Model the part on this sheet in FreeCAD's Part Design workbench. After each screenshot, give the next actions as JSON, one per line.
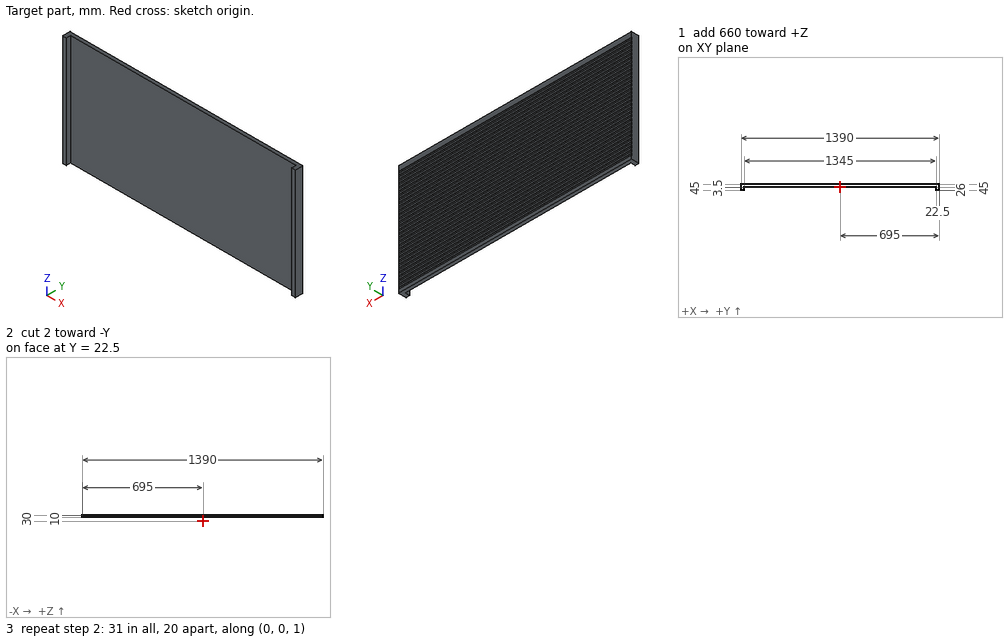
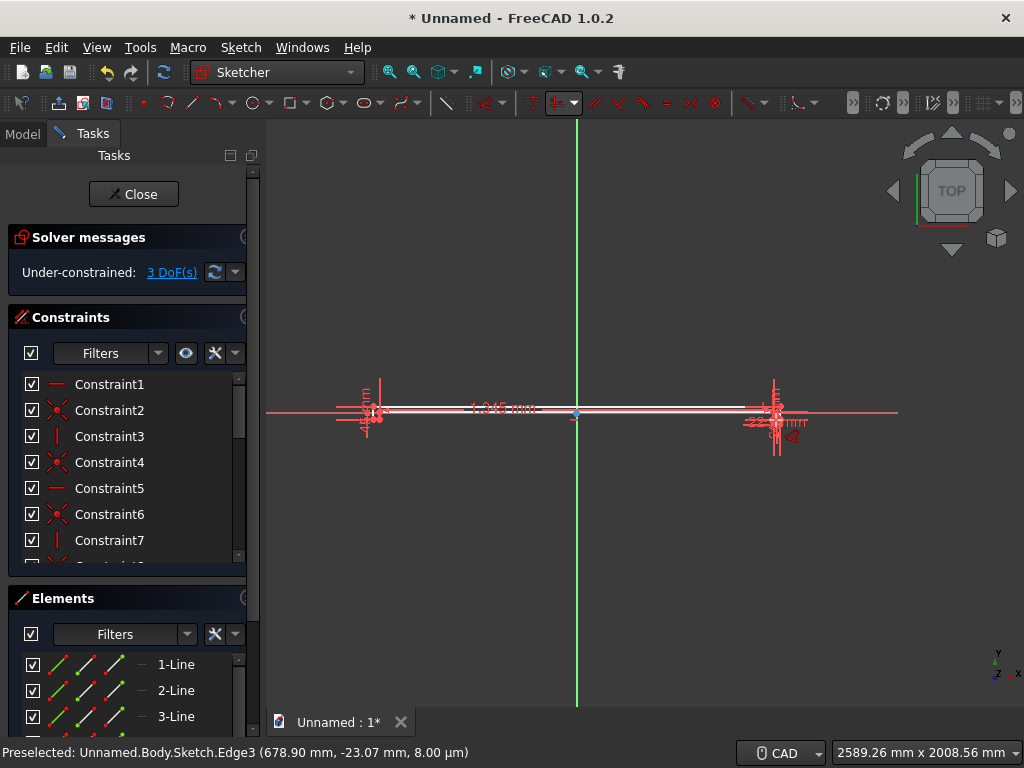
{"action": "scroll", "coordinate": [658, 407], "scroll_direction": "up", "scroll_amount": 5}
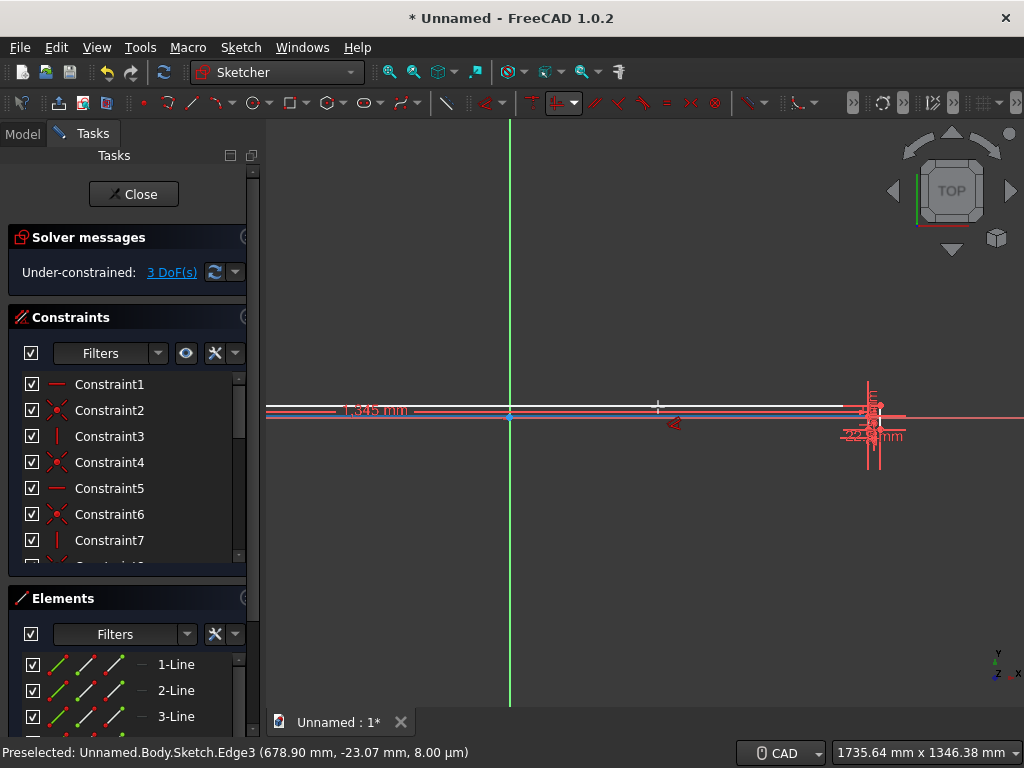
{"action": "left_click", "coordinate": [657, 405]}
{"action": "left_click", "coordinate": [576, 371]}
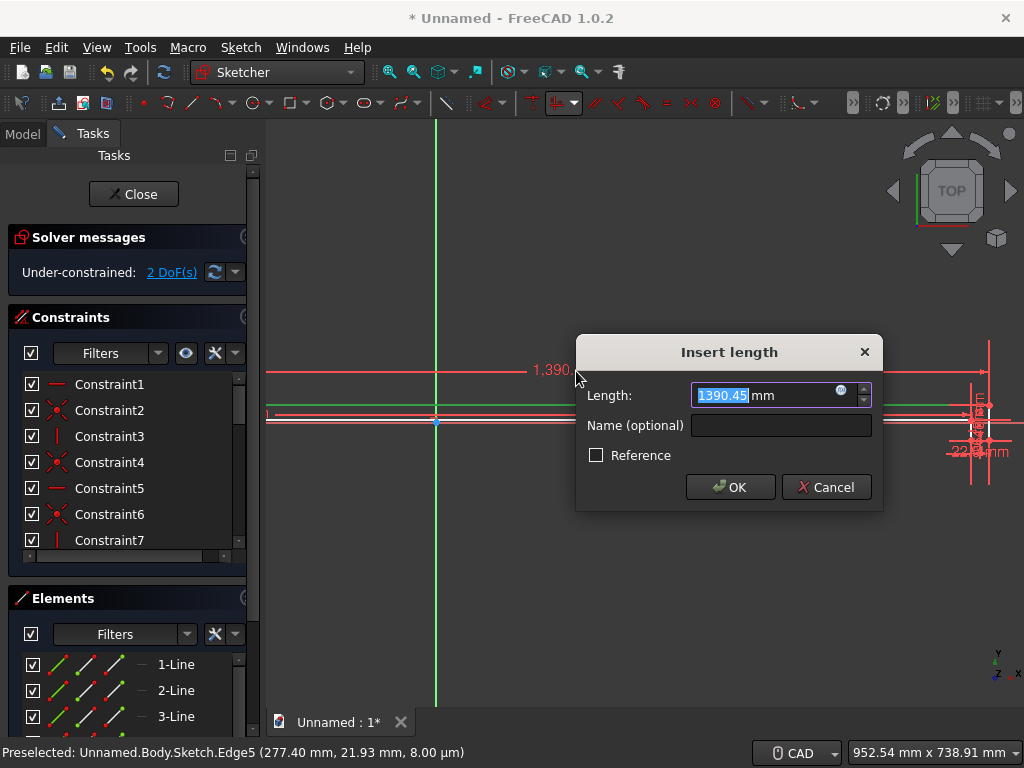
{"action": "type", "text": "1390"}
{"action": "key", "text": "Return"}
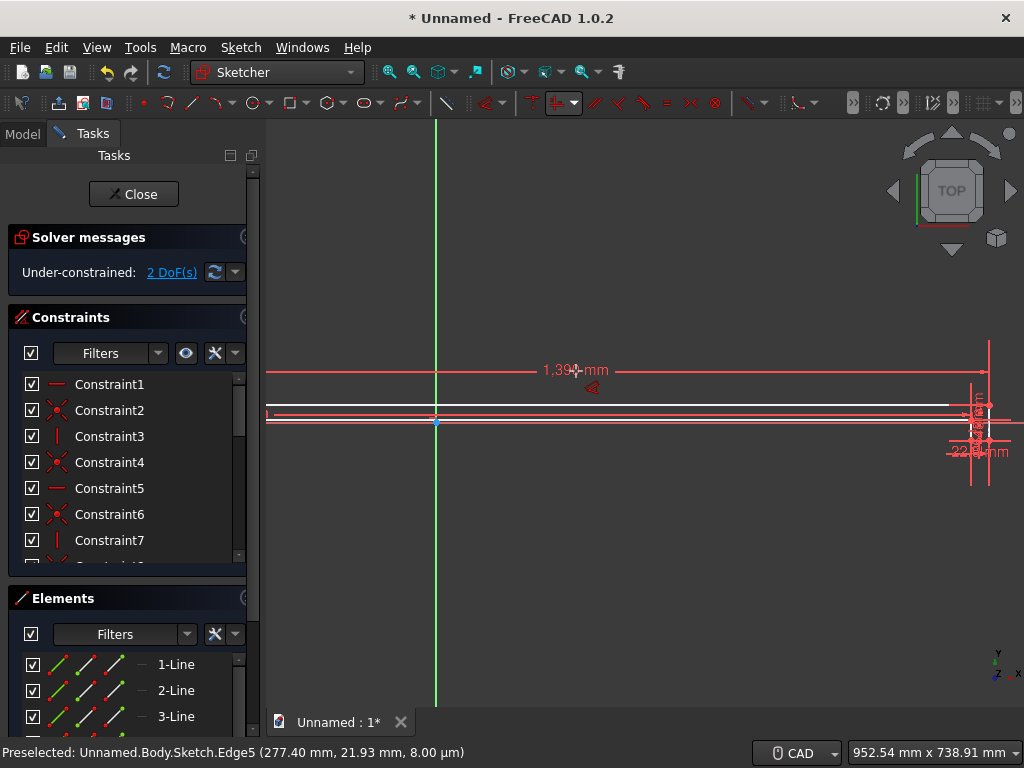
{"action": "scroll", "coordinate": [658, 407], "scroll_direction": "down", "scroll_amount": 5}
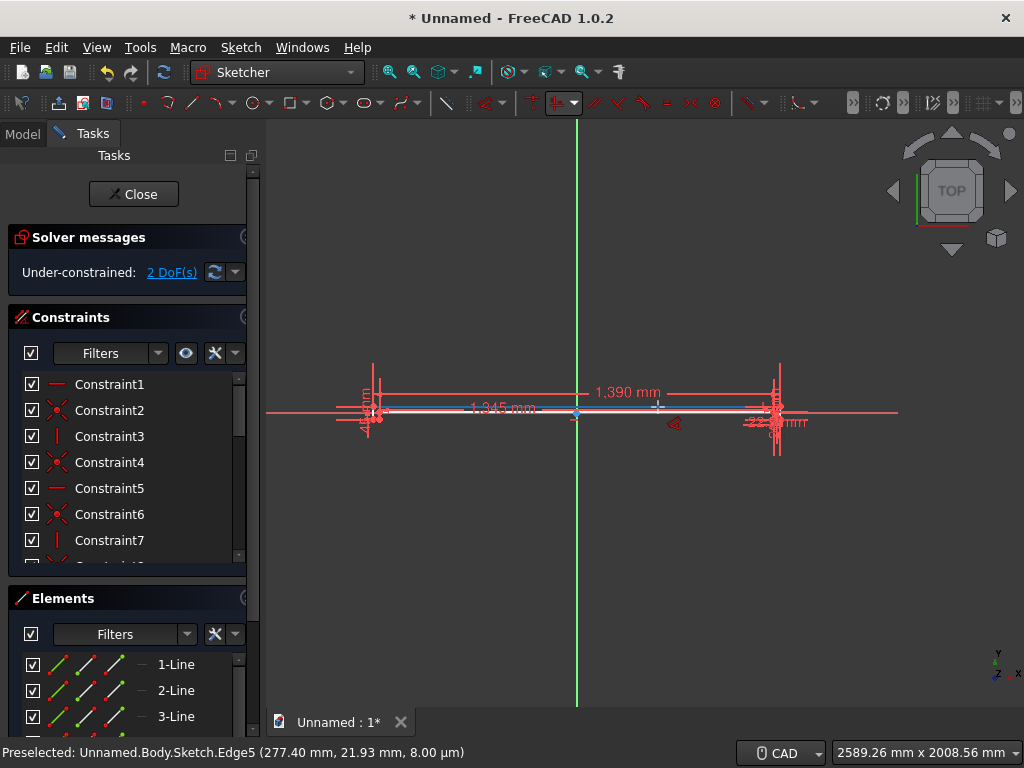
{"action": "scroll", "coordinate": [380, 412], "scroll_direction": "up", "scroll_amount": 19}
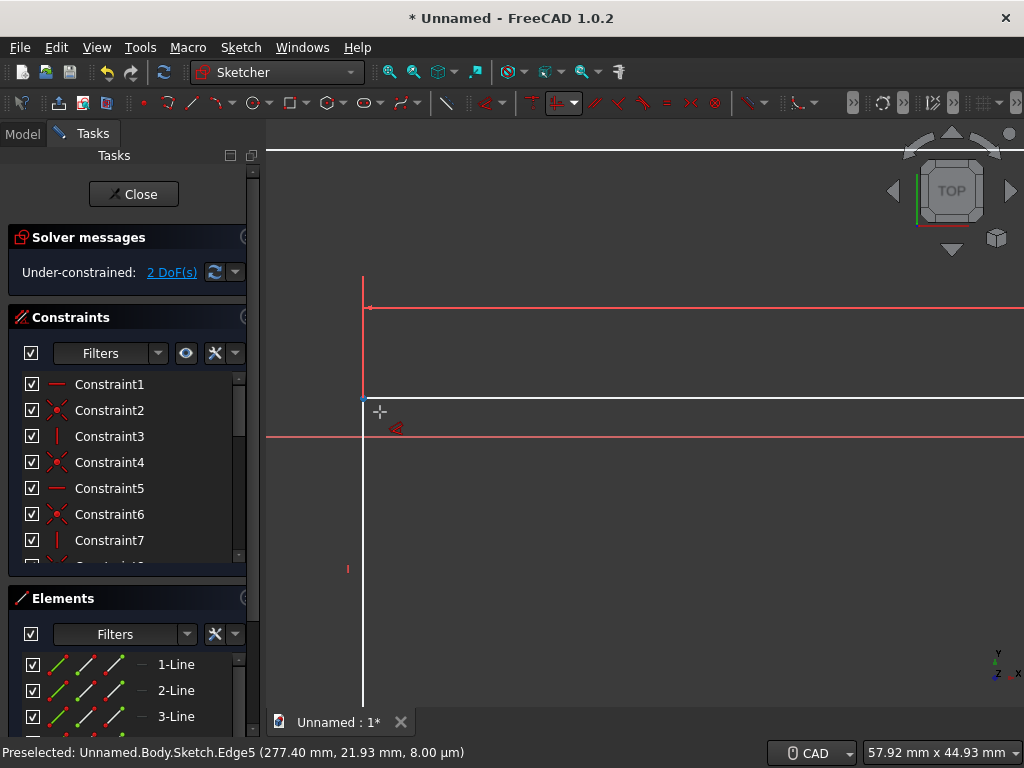
{"action": "left_click", "coordinate": [363, 398]}
{"action": "left_click", "coordinate": [329, 417]}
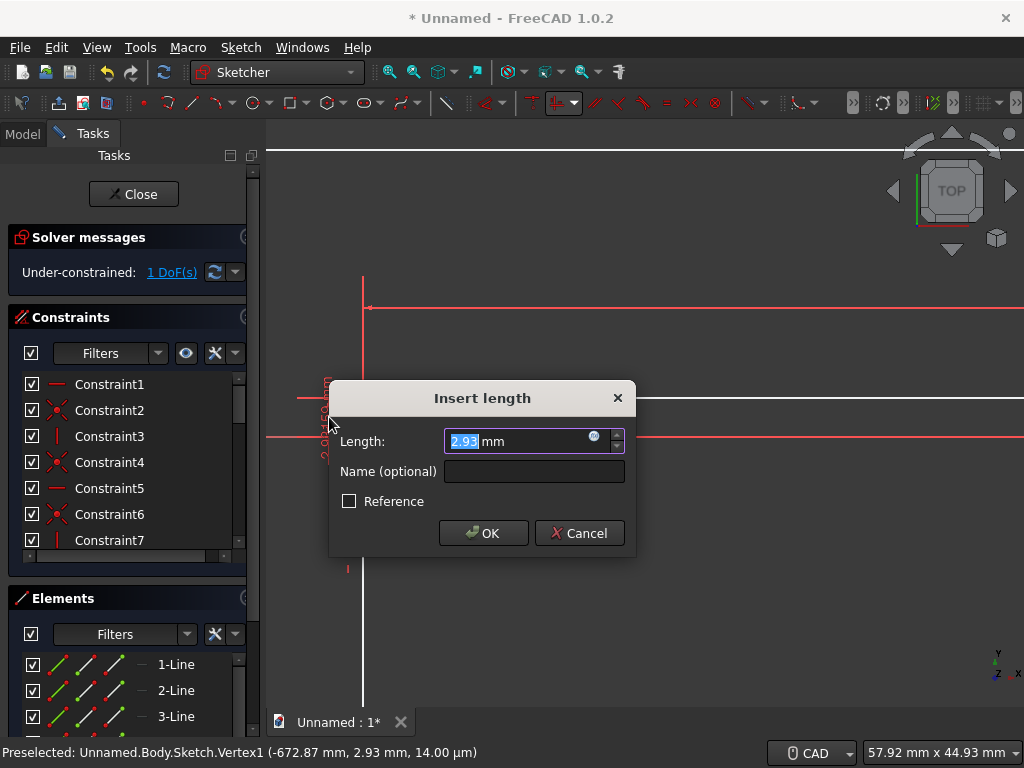
{"action": "type", "text": "3.5"}
{"action": "key", "text": "Return"}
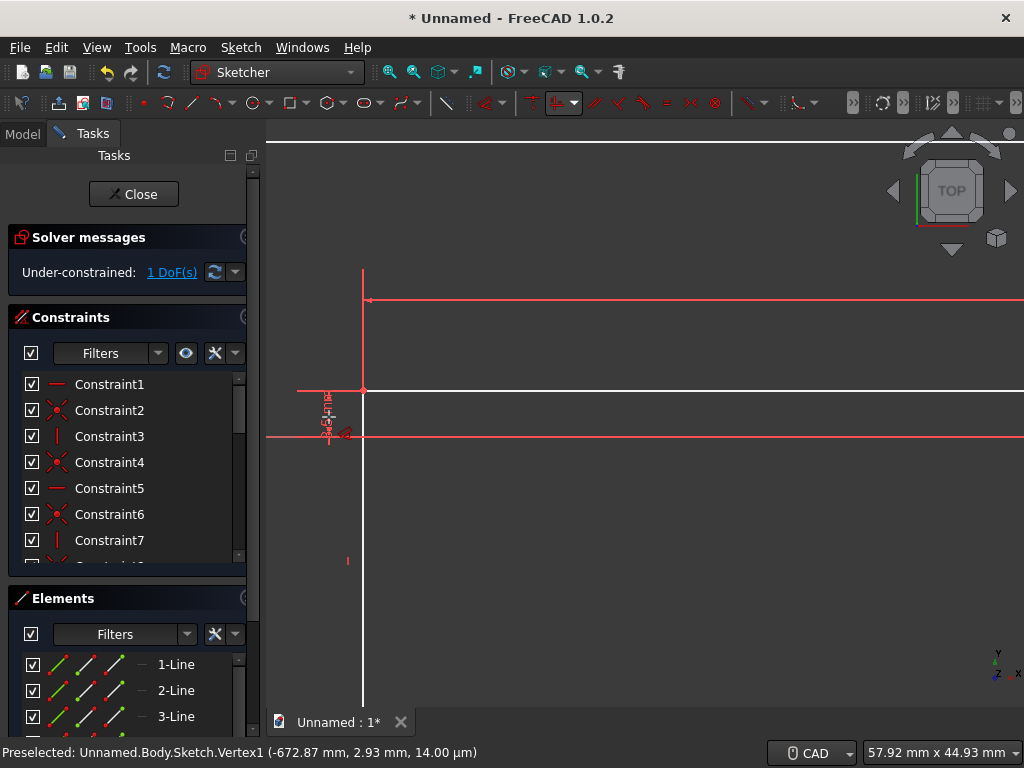
{"action": "scroll", "coordinate": [335, 412], "scroll_direction": "down", "scroll_amount": 18}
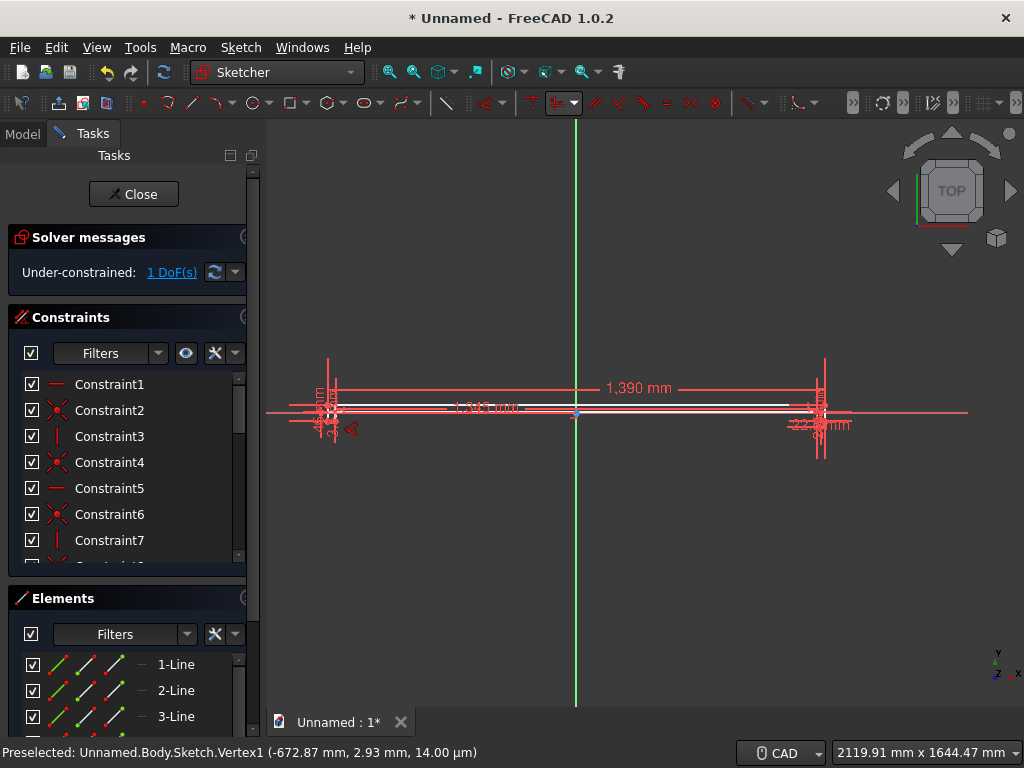
{"action": "scroll", "coordinate": [825, 421], "scroll_direction": "up", "scroll_amount": 3}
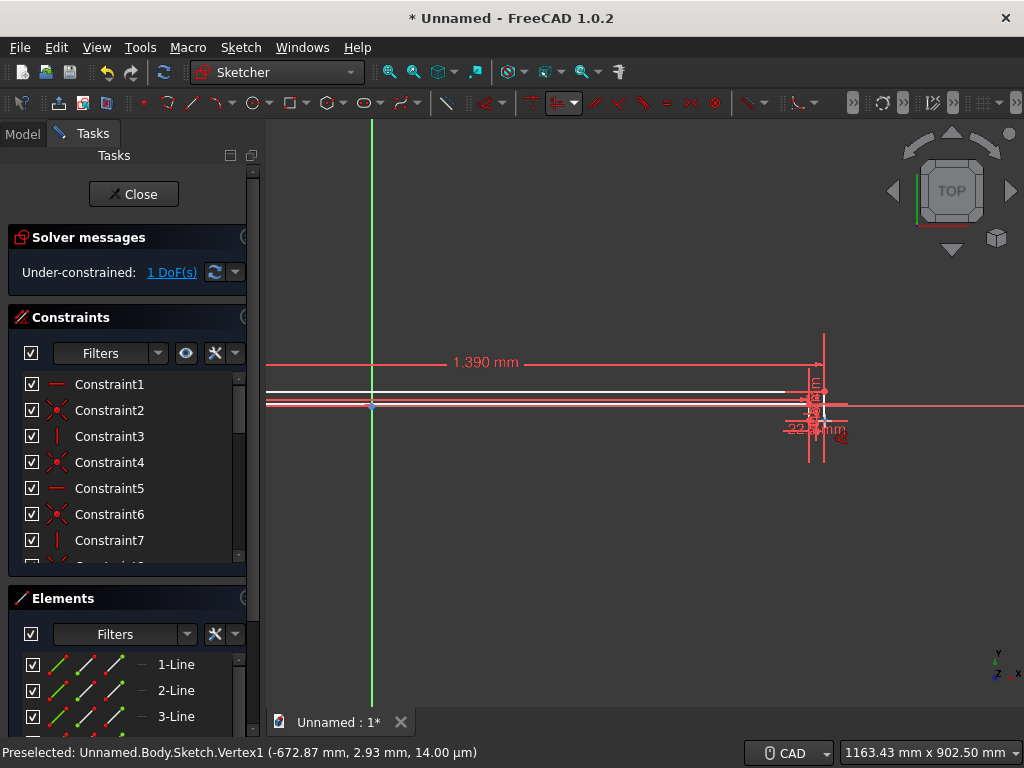
{"action": "left_click", "coordinate": [824, 421]}
{"action": "left_click", "coordinate": [598, 455]}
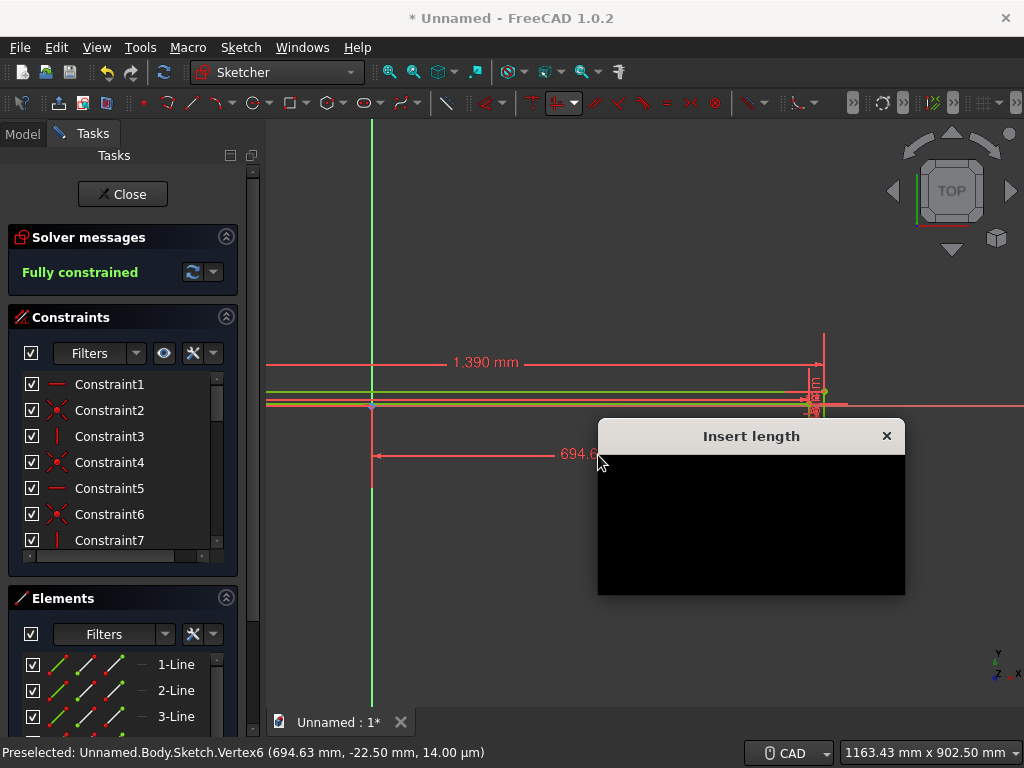
{"action": "type", "text": "695"}
{"action": "key", "text": "Return"}
{"action": "key", "text": "Escape"}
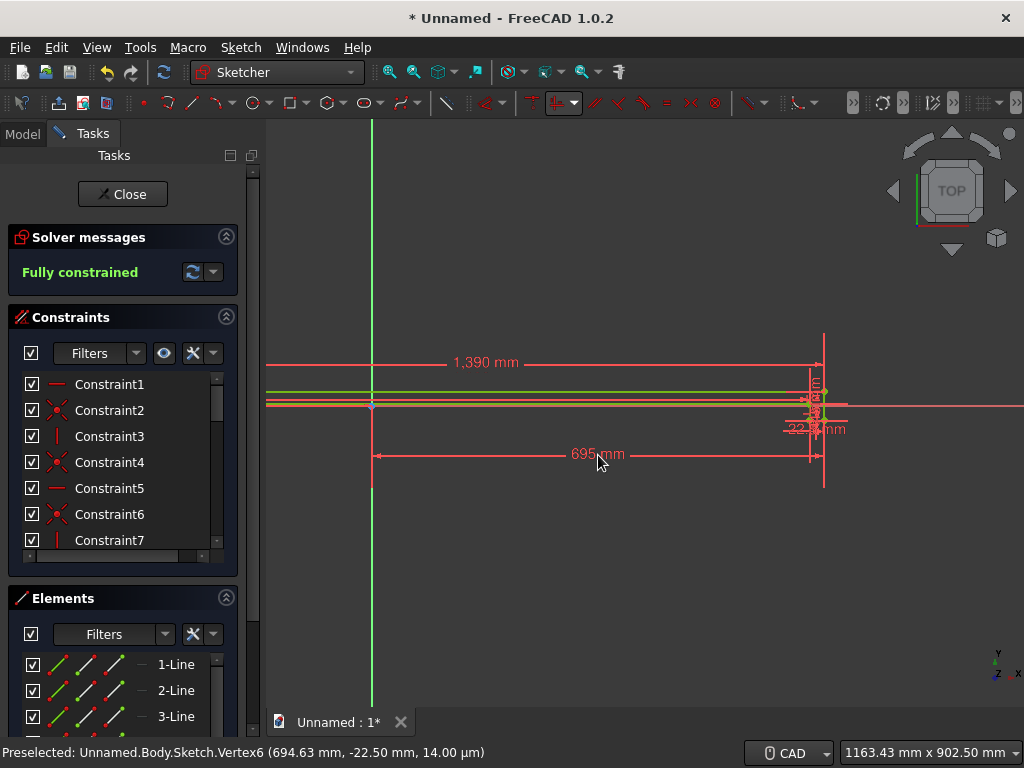
{"action": "left_click", "coordinate": [123, 194]}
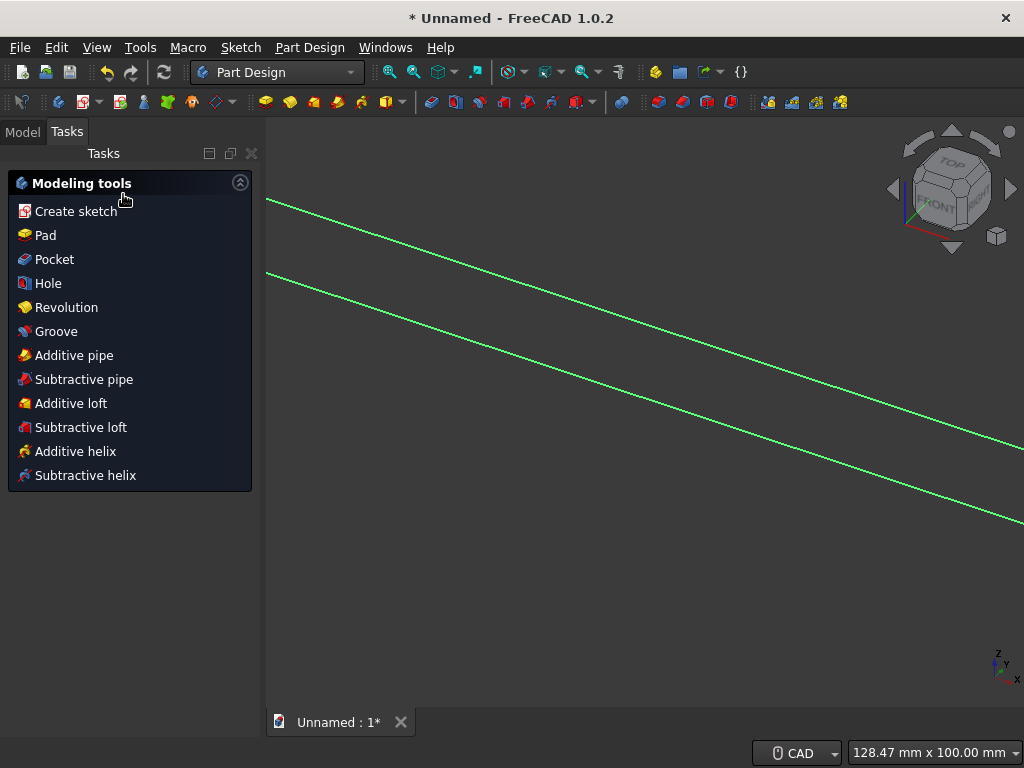
{"action": "left_click", "coordinate": [266, 102]}